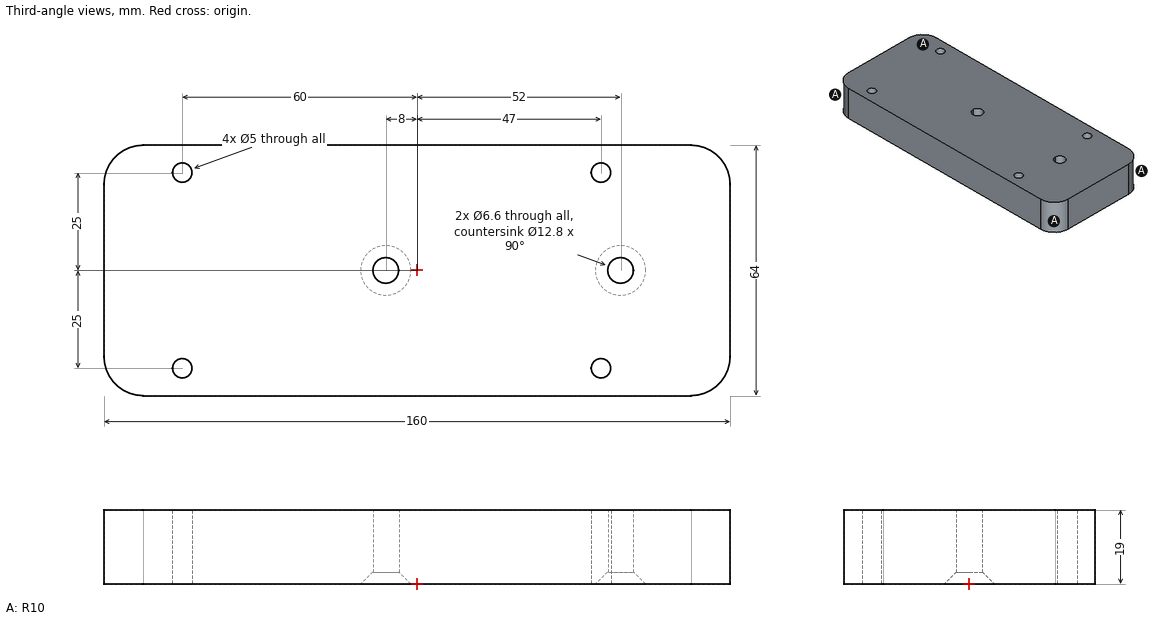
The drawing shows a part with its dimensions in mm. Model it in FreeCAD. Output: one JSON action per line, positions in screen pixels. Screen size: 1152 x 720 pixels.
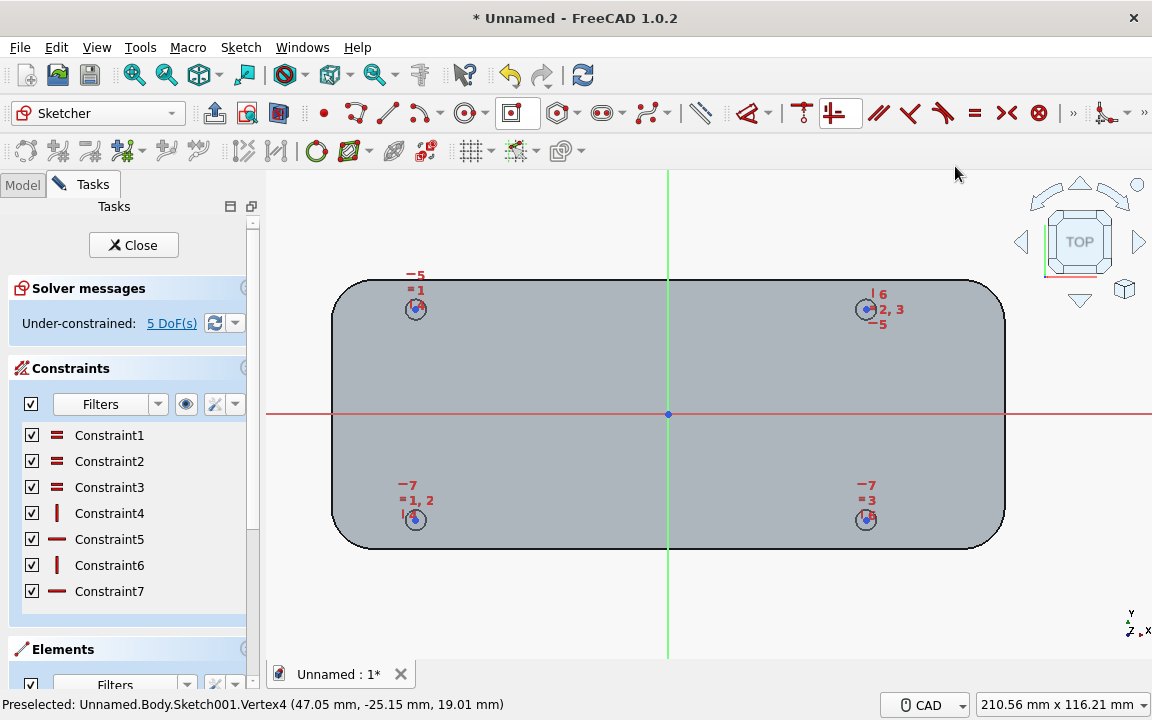
{"action": "left_click", "coordinate": [748, 114]}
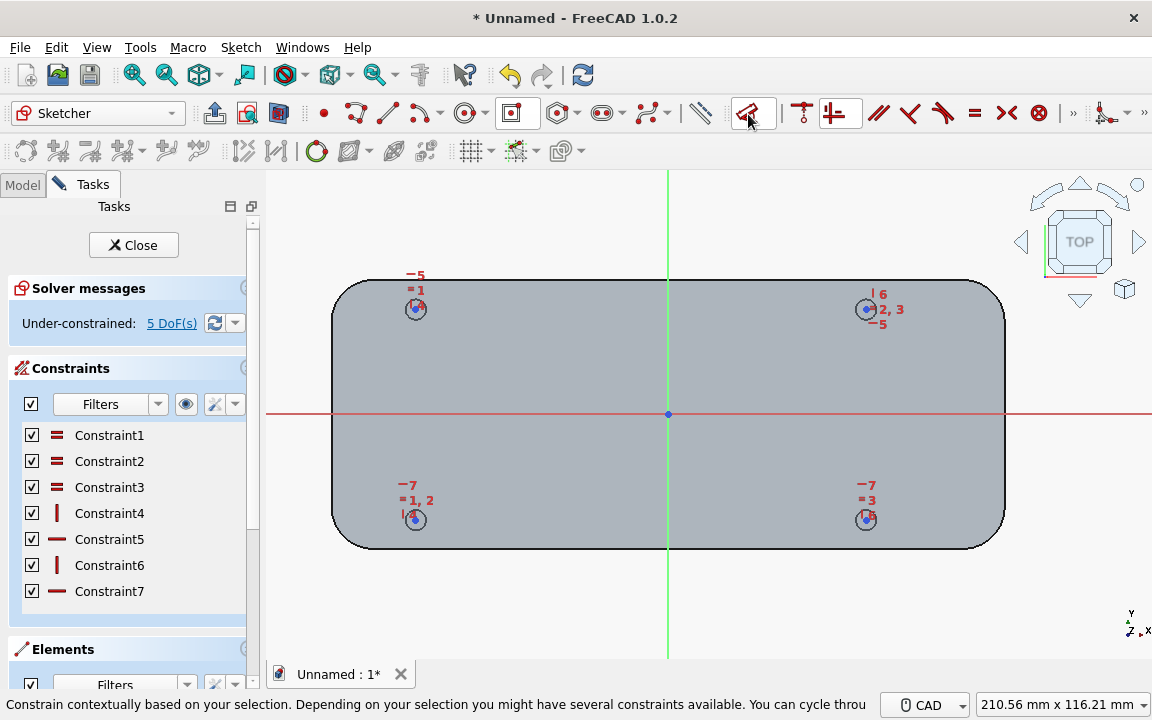
{"action": "scroll", "coordinate": [423, 302], "scroll_direction": "up", "scroll_amount": 4}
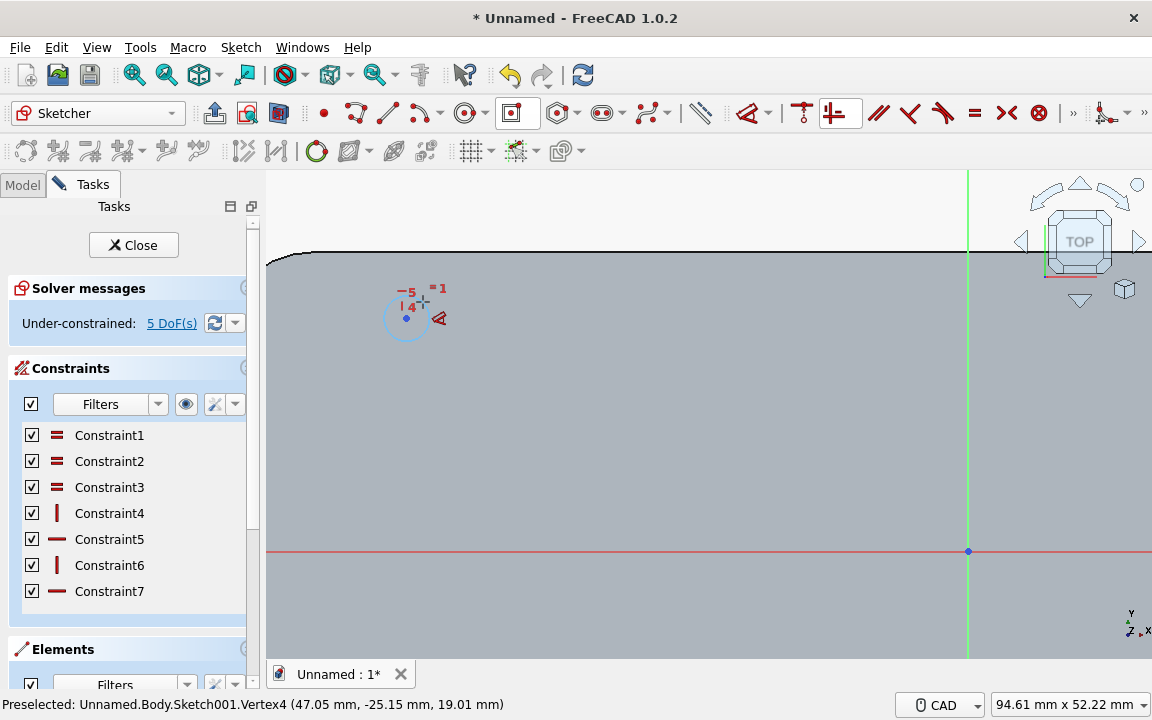
{"action": "left_click", "coordinate": [423, 303]}
{"action": "left_click", "coordinate": [446, 281]}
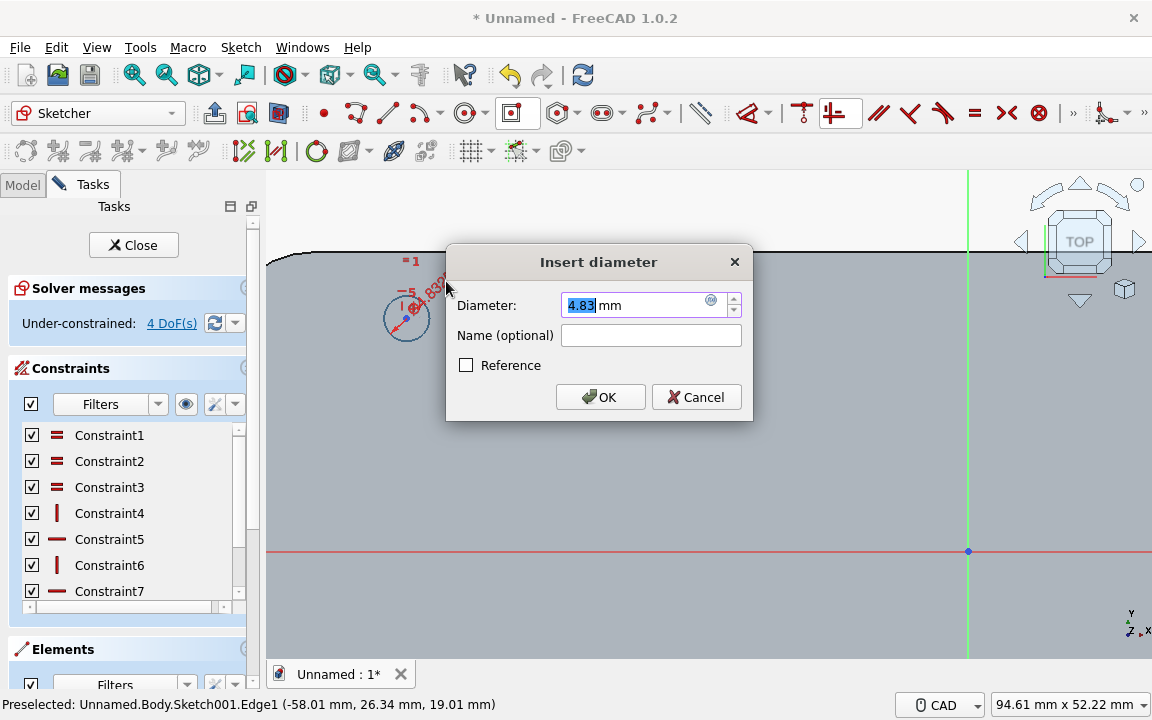
{"action": "type", "text": "5"}
{"action": "key", "text": "Return"}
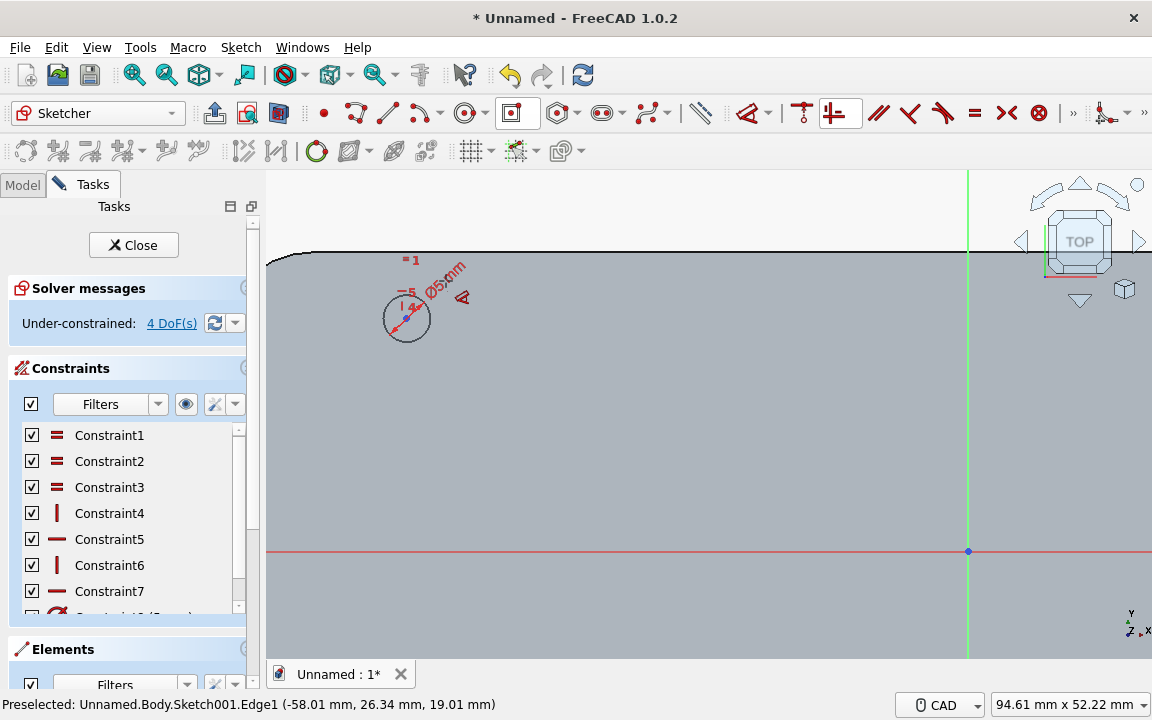
{"action": "left_click", "coordinate": [407, 319]}
{"action": "left_click", "coordinate": [688, 285]}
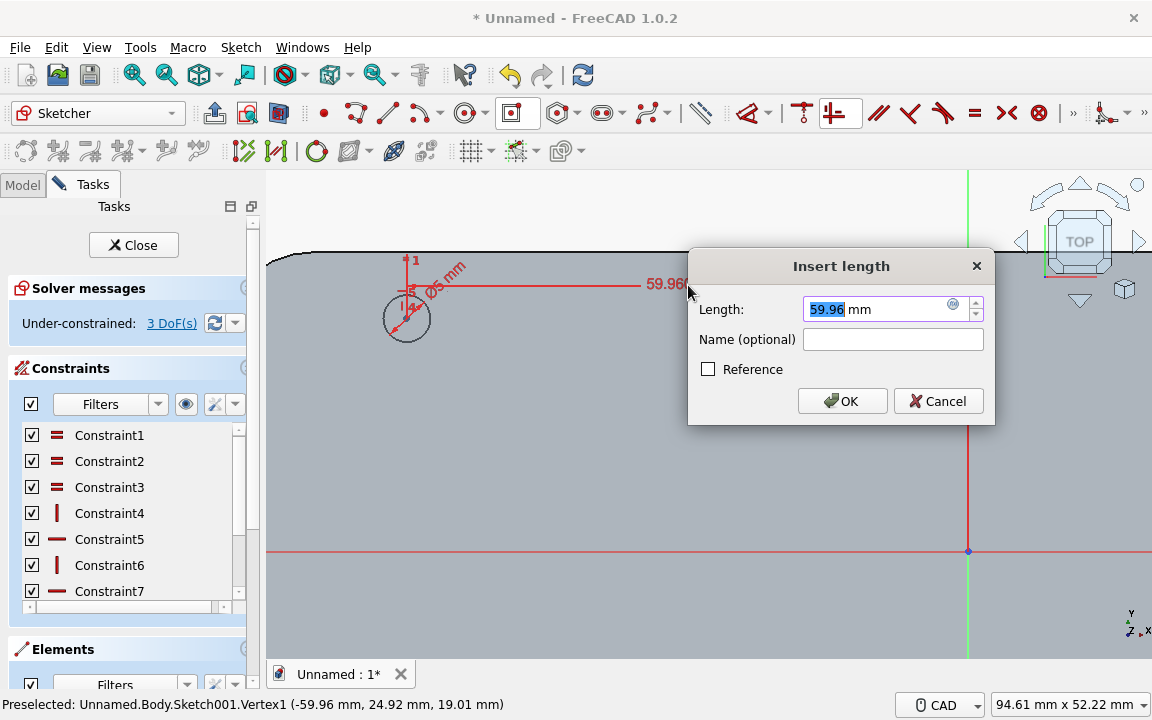
{"action": "type", "text": "60"}
{"action": "key", "text": "Return"}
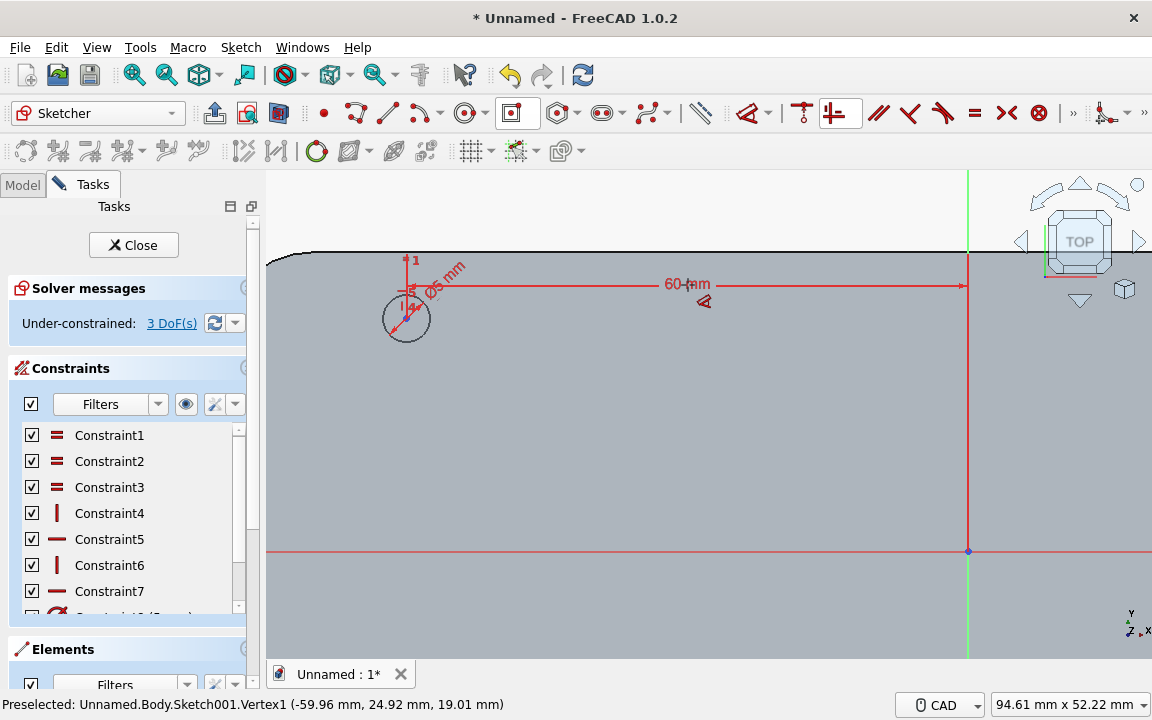
{"action": "left_click", "coordinate": [407, 319]}
{"action": "left_click", "coordinate": [373, 435]}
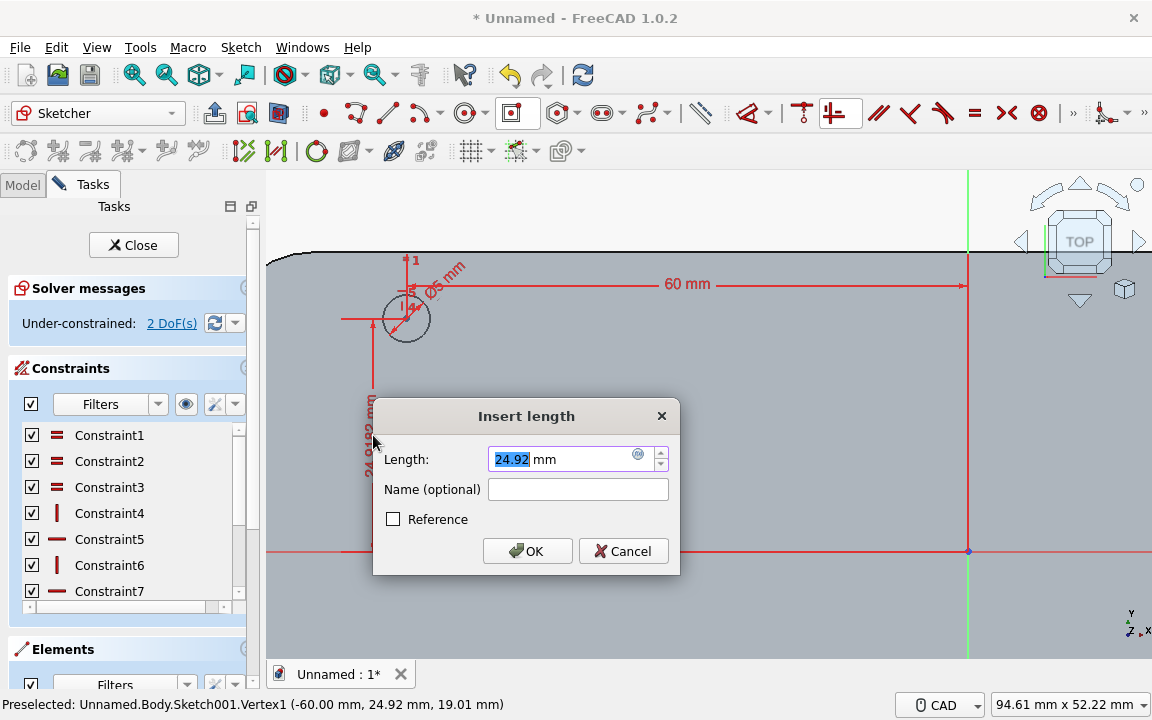
{"action": "type", "text": "25"}
{"action": "key", "text": "Return"}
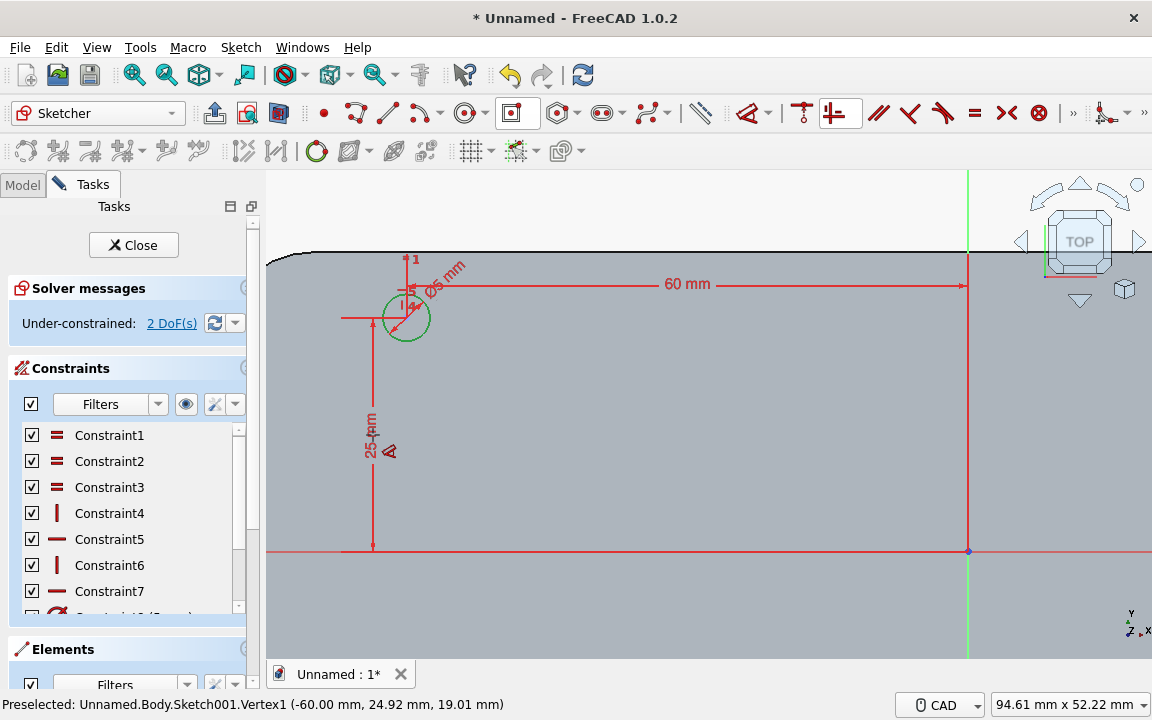
{"action": "scroll", "coordinate": [423, 302], "scroll_direction": "down", "scroll_amount": 4}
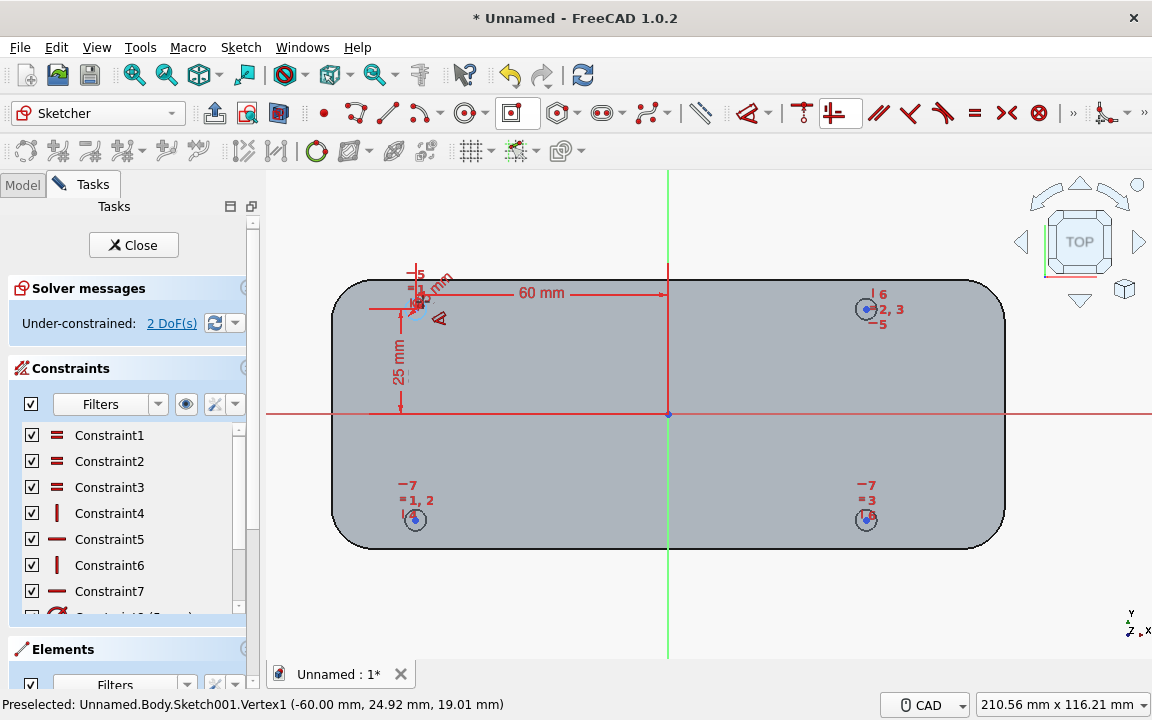
{"action": "left_click", "coordinate": [416, 520]}
{"action": "left_click", "coordinate": [382, 467]}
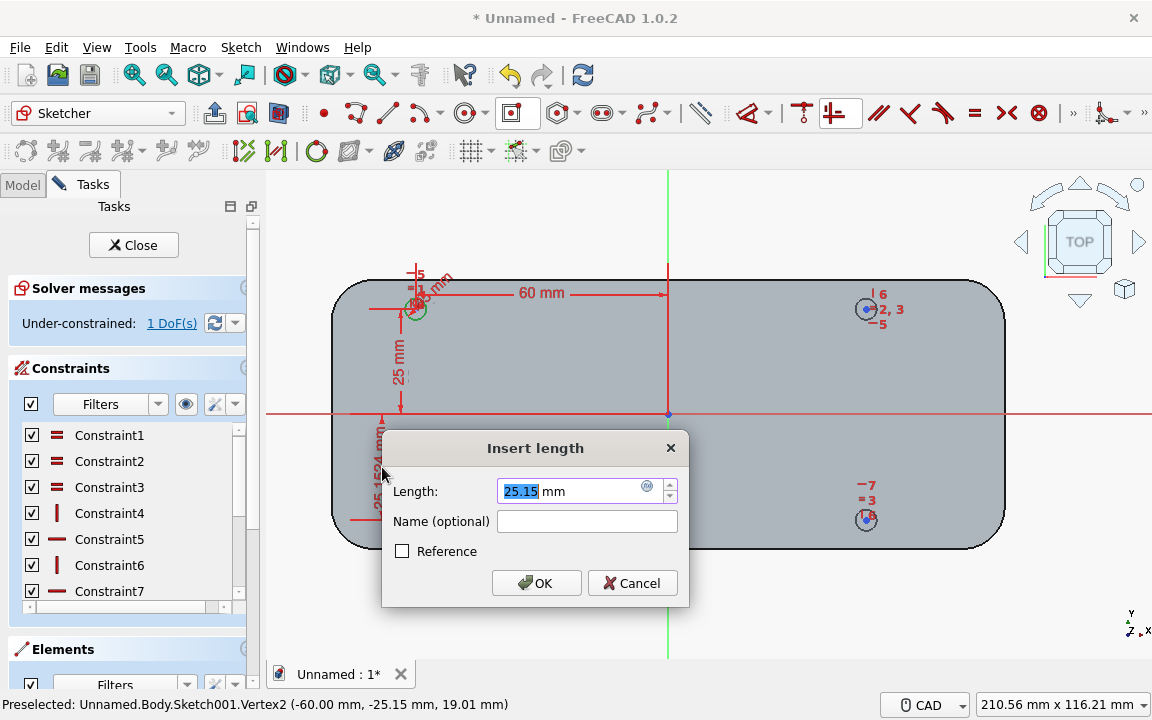
{"action": "type", "text": "25"}
{"action": "key", "text": "Return"}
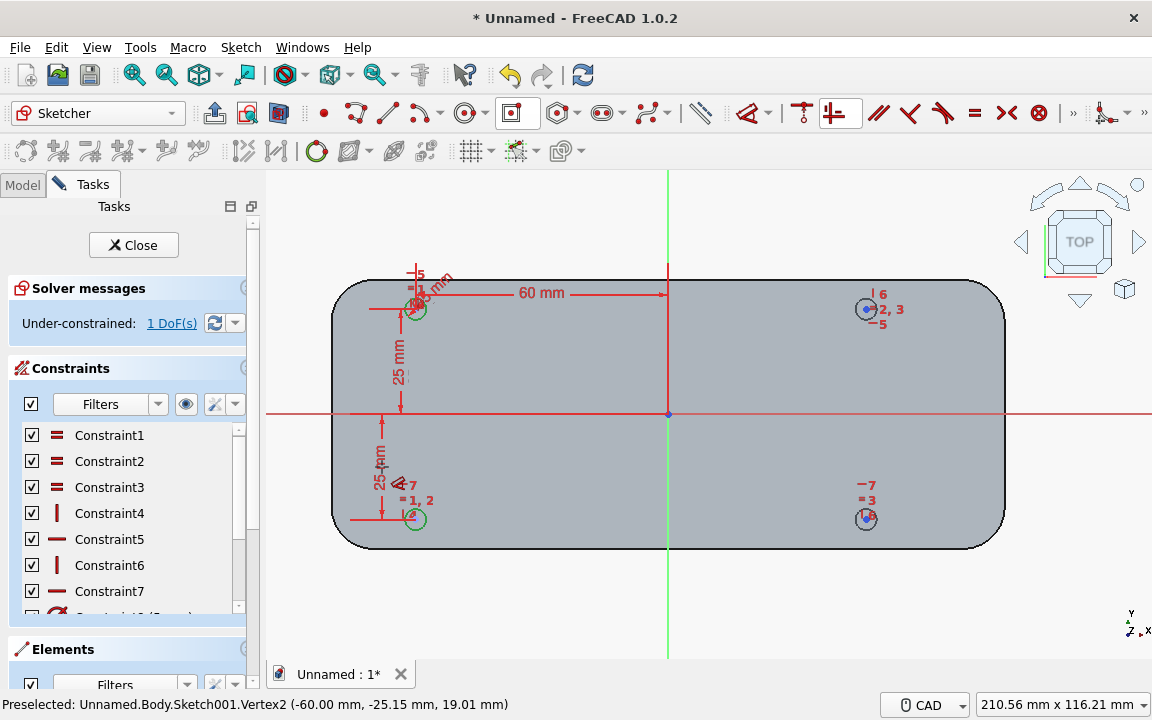
{"action": "left_click", "coordinate": [866, 309]}
{"action": "left_click", "coordinate": [767, 275]}